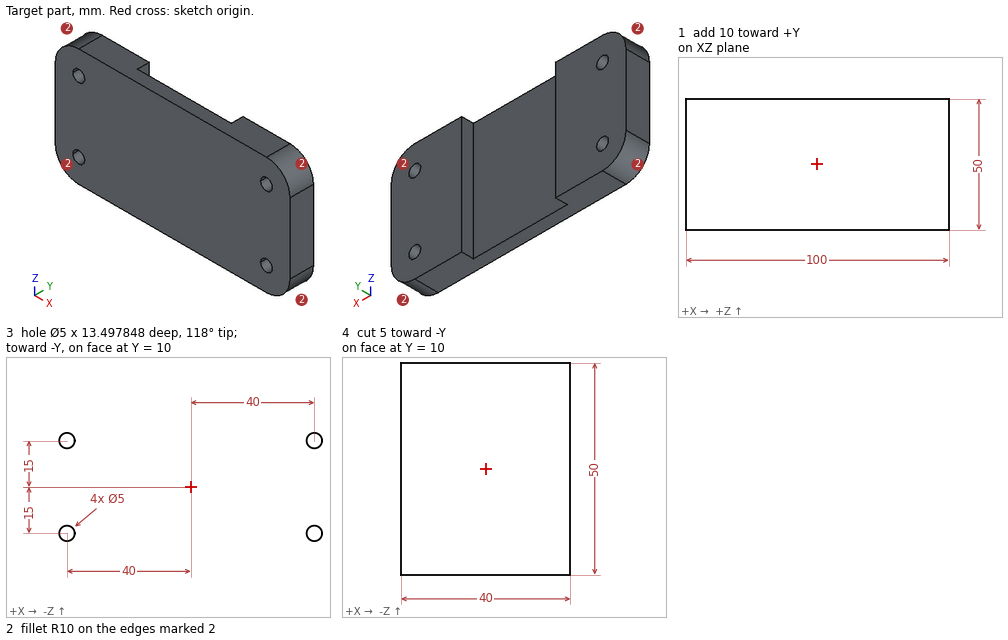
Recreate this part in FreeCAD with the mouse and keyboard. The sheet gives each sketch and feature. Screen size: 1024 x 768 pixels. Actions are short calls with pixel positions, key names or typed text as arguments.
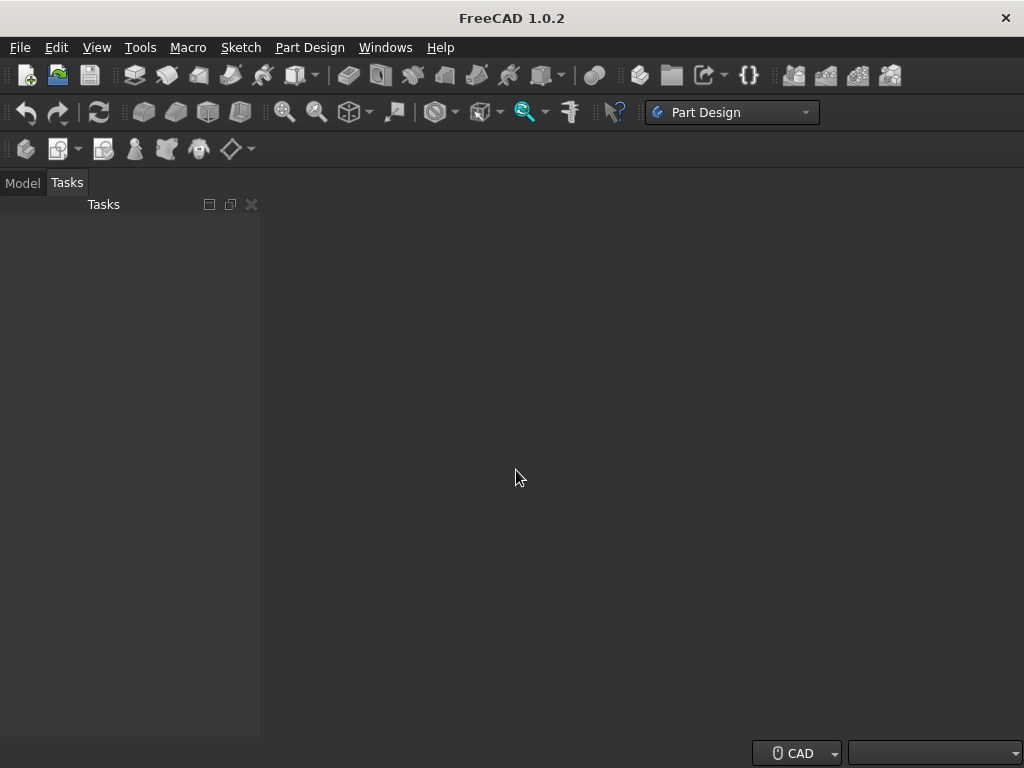
key(ctrl+n)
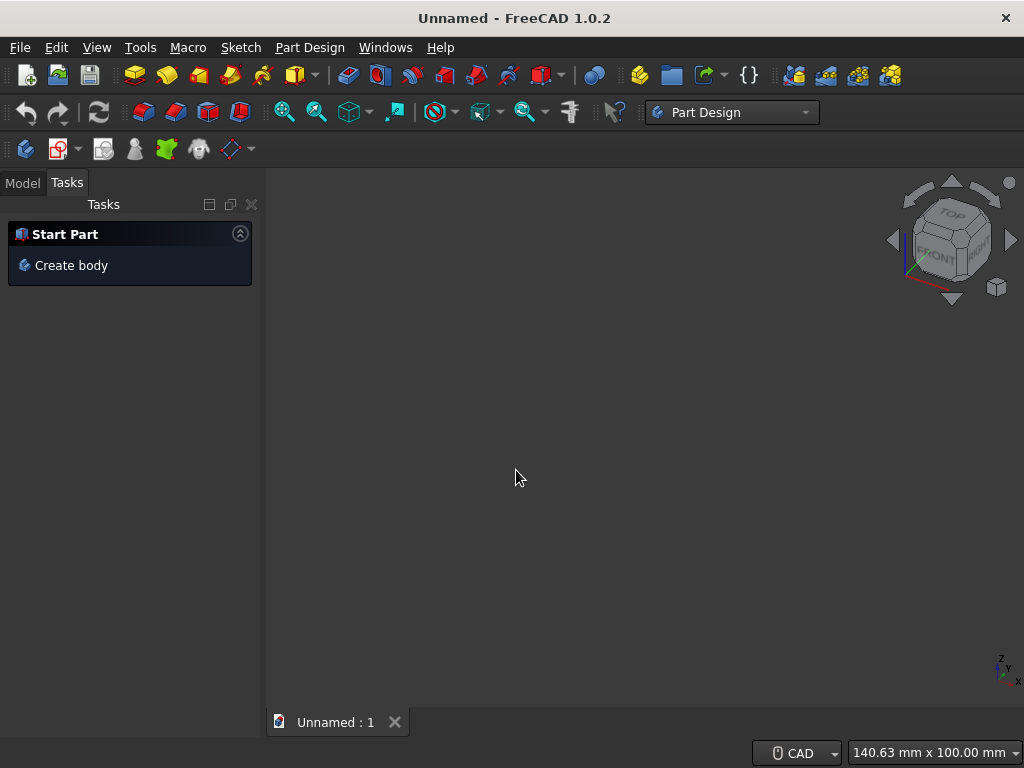
click(58, 150)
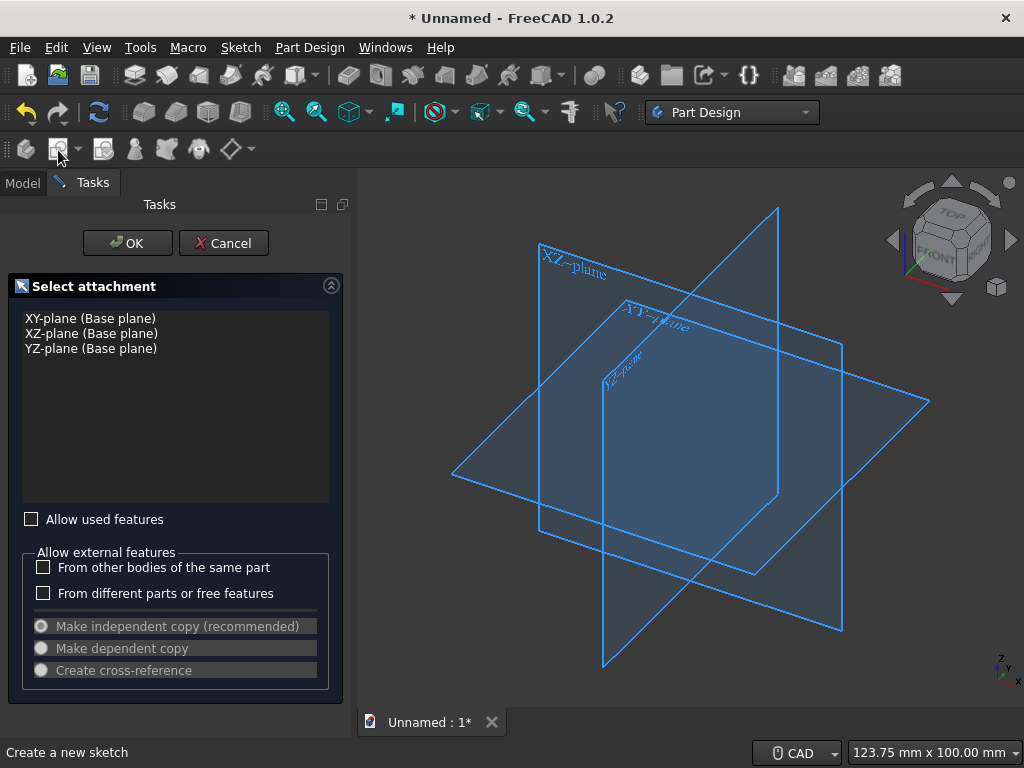
click(82, 334)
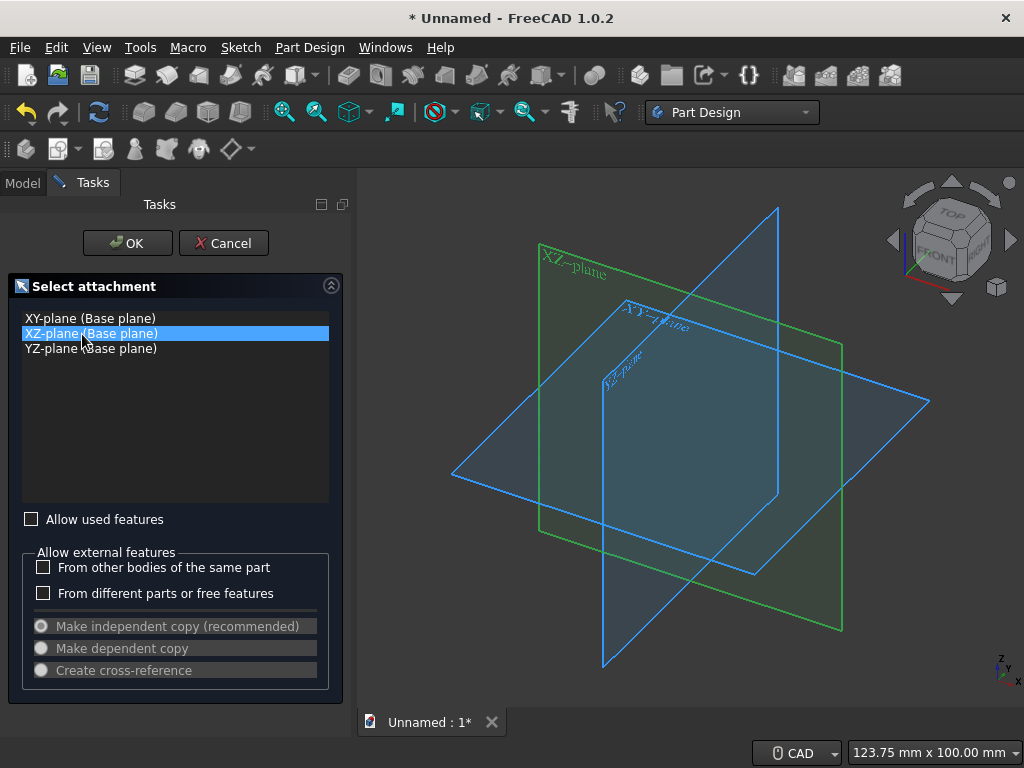
click(128, 243)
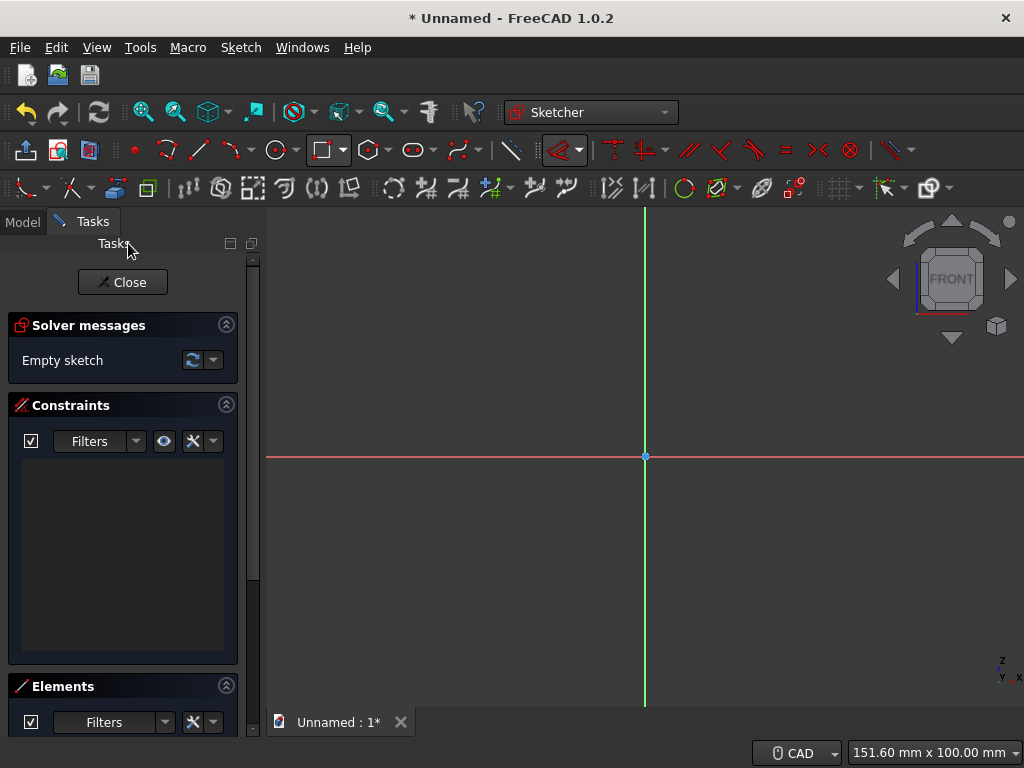
scroll(294, 457, down, 1)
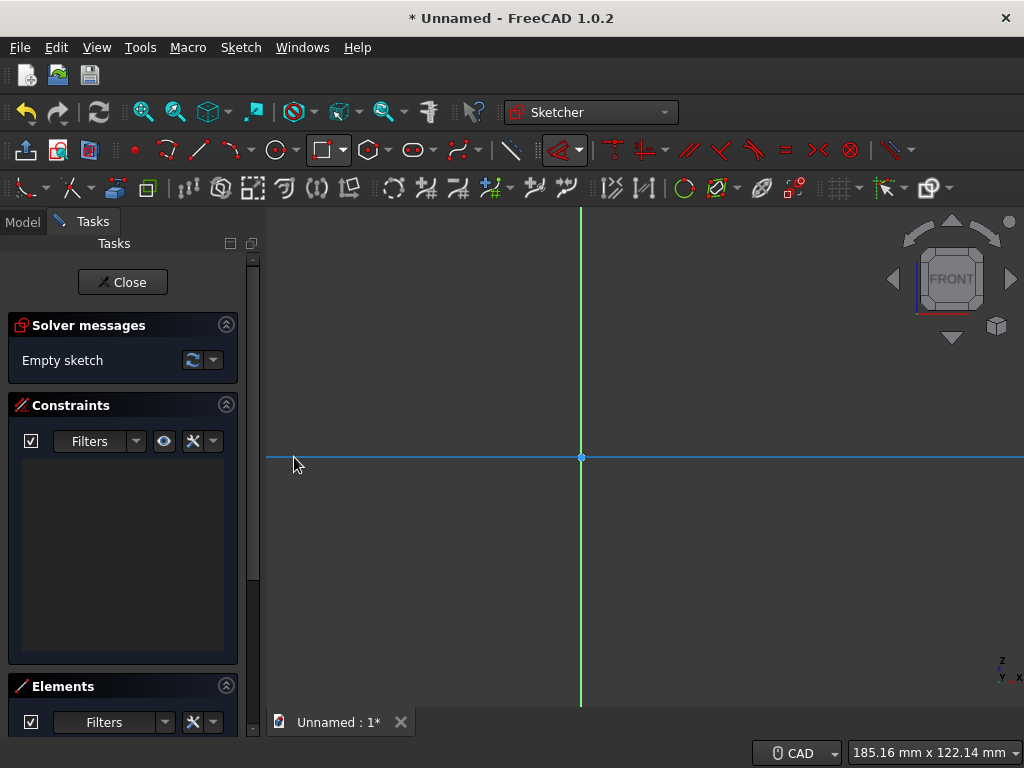
click(346, 150)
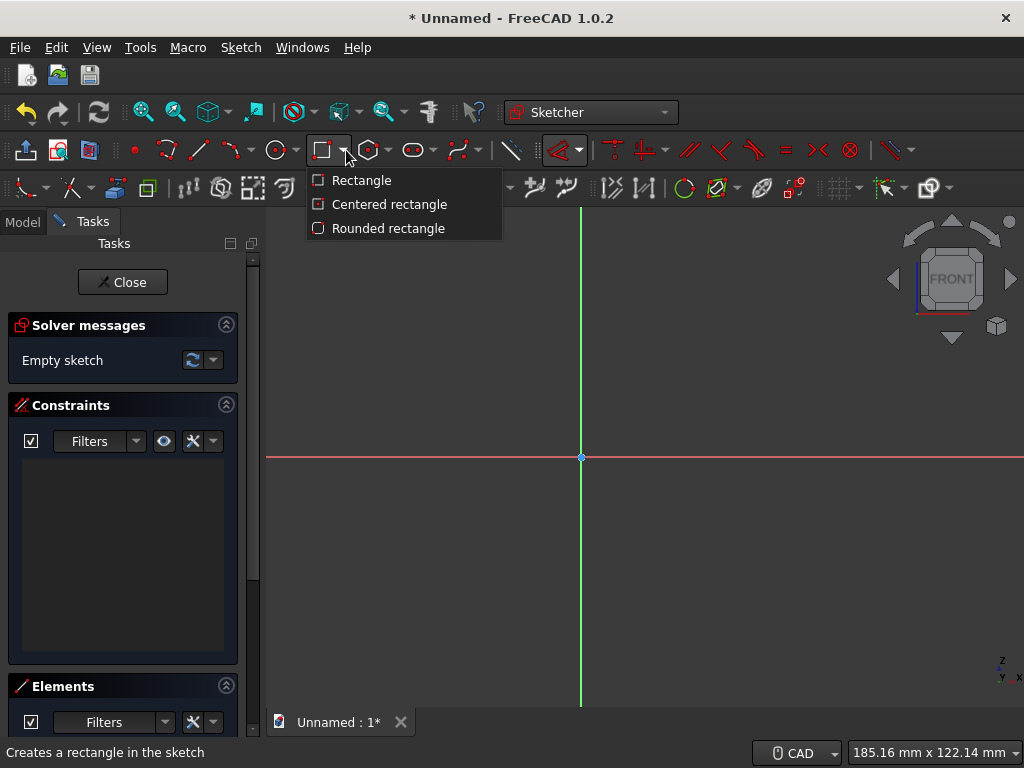
click(404, 204)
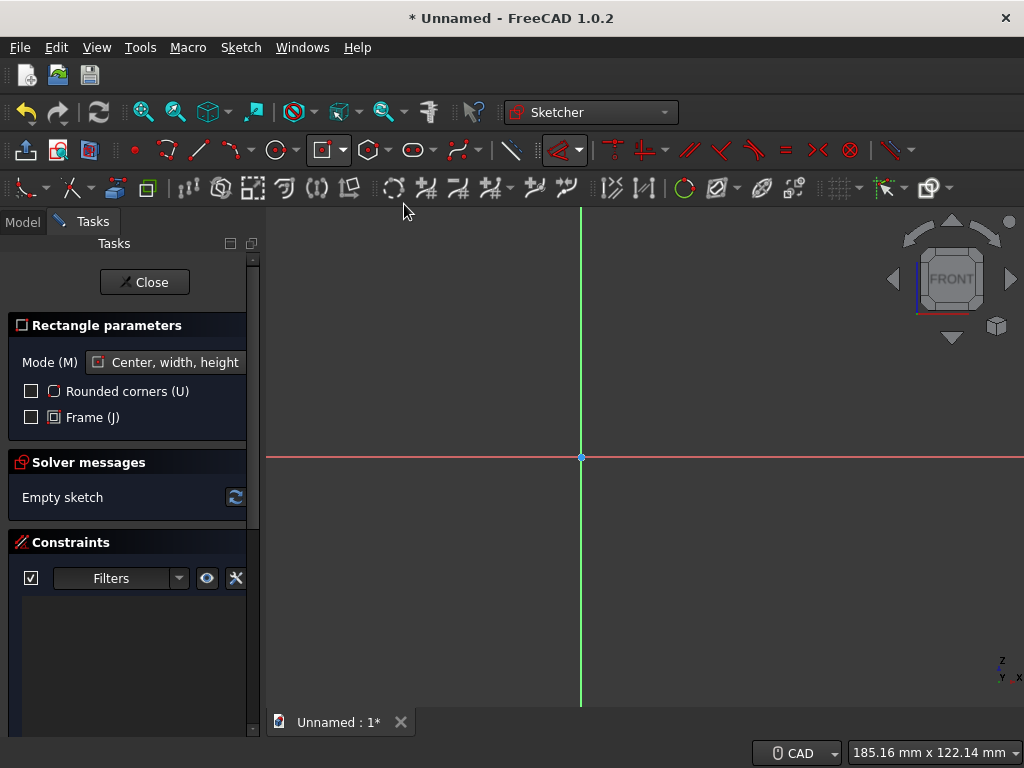
click(581, 457)
move(786, 355)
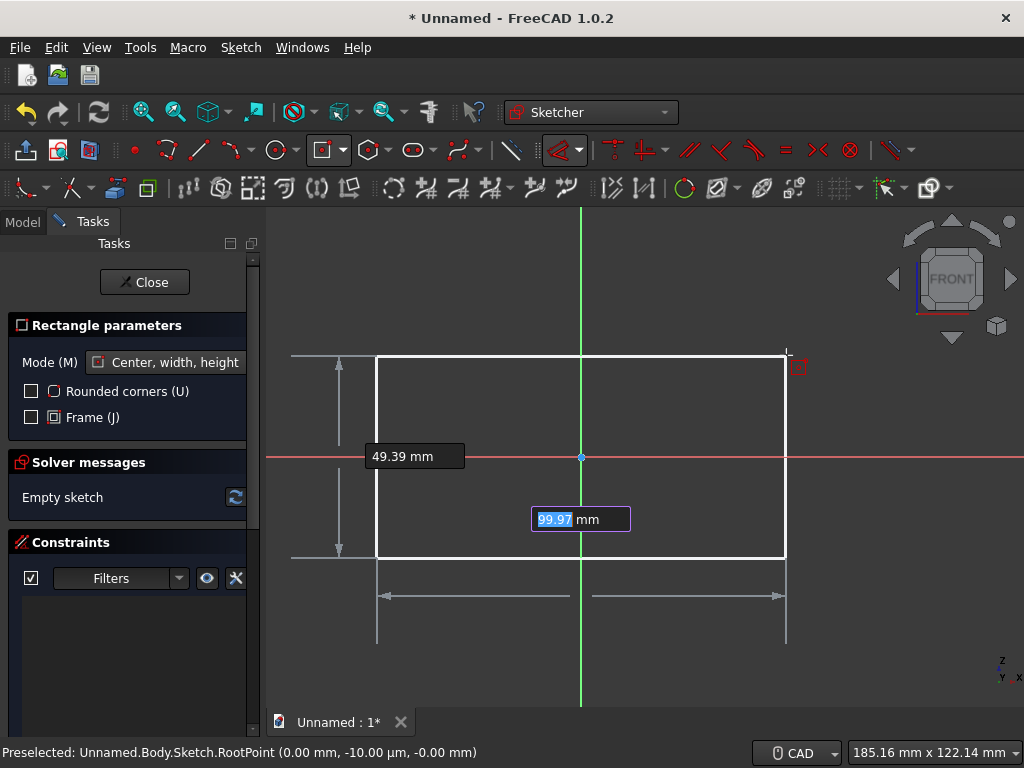
text(100)
key(Tab)
text(50)
key(Return)
key(Escape)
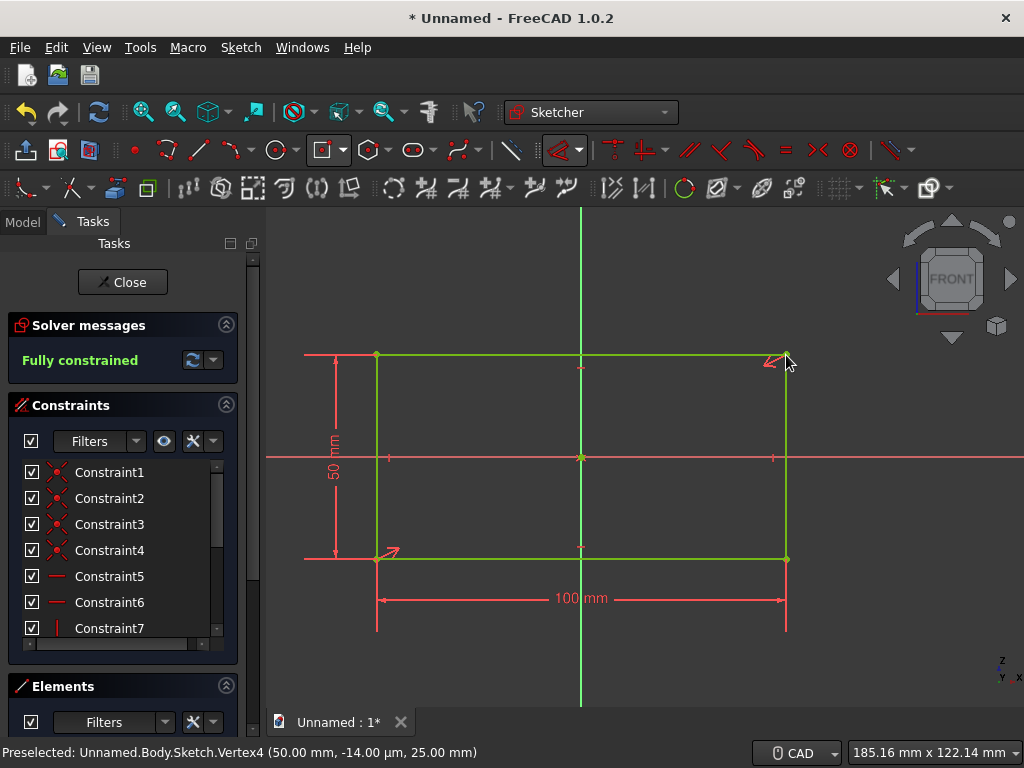
click(123, 282)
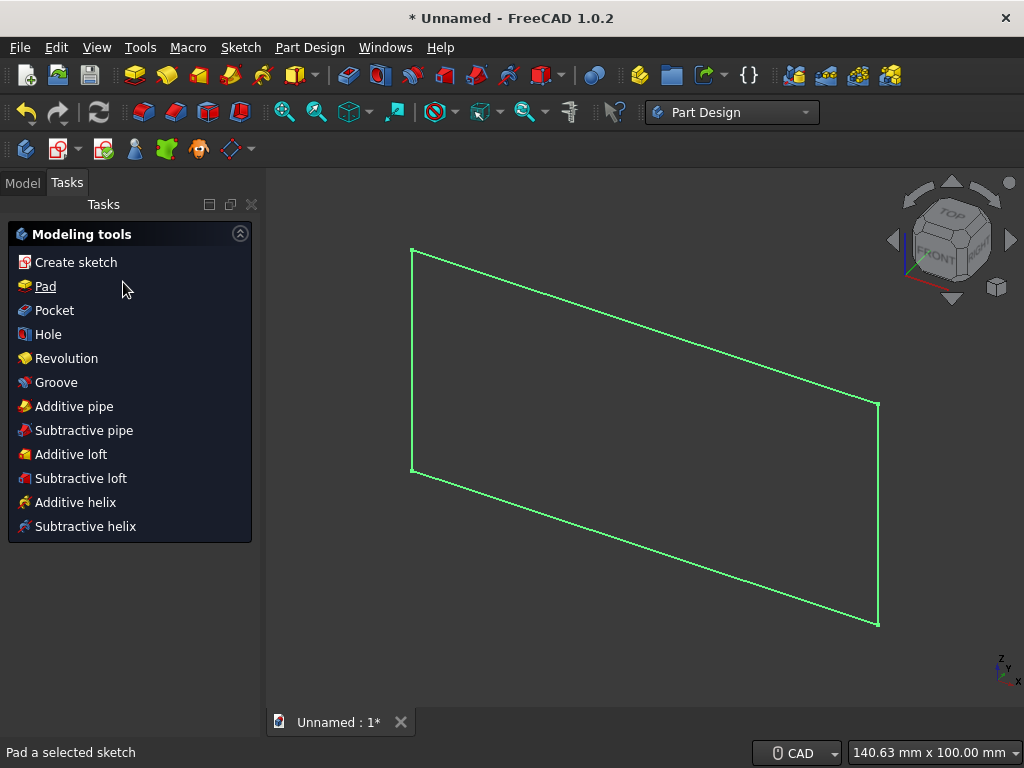
click(136, 76)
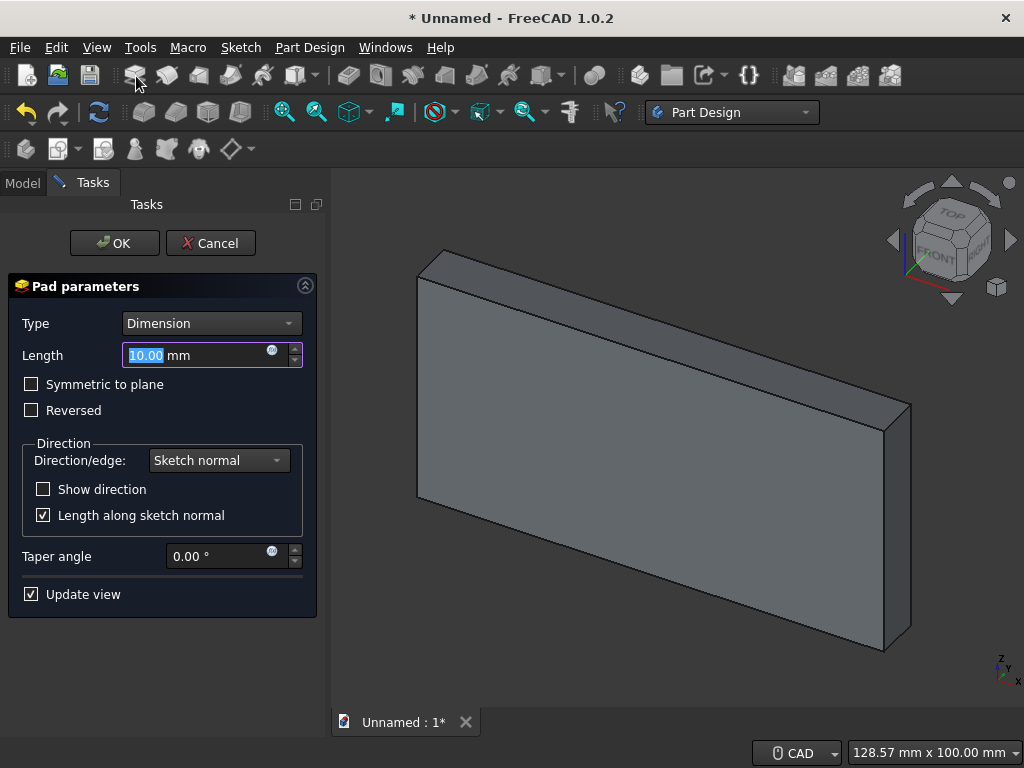
text(10)
key(Tab)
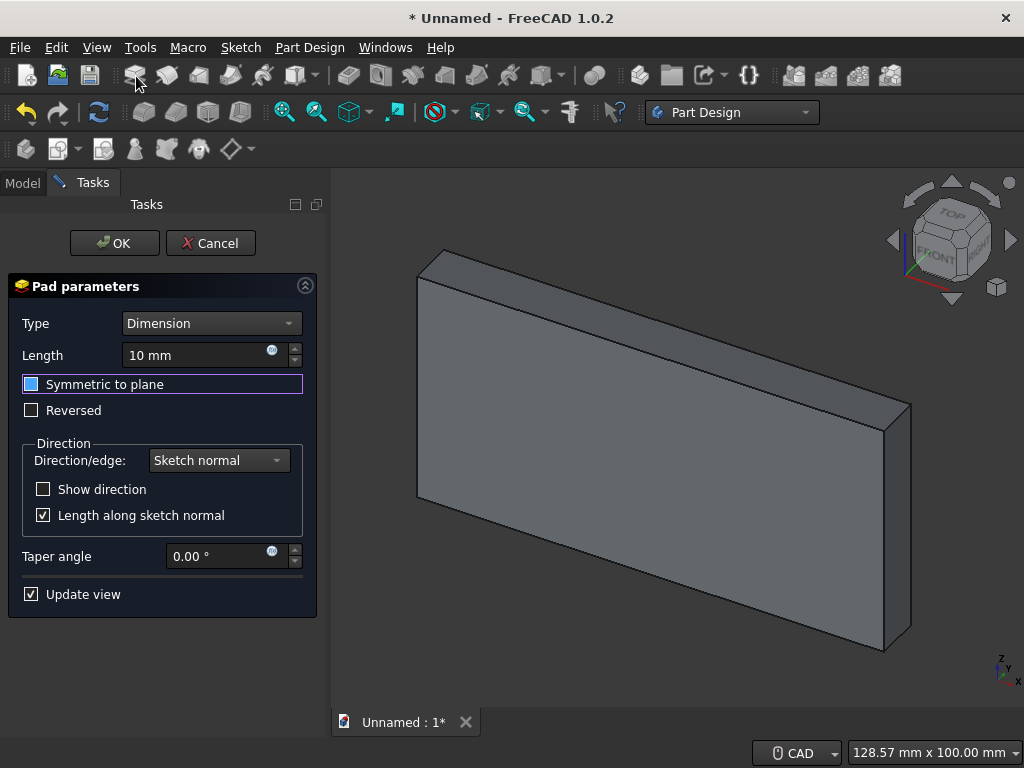
click(30, 410)